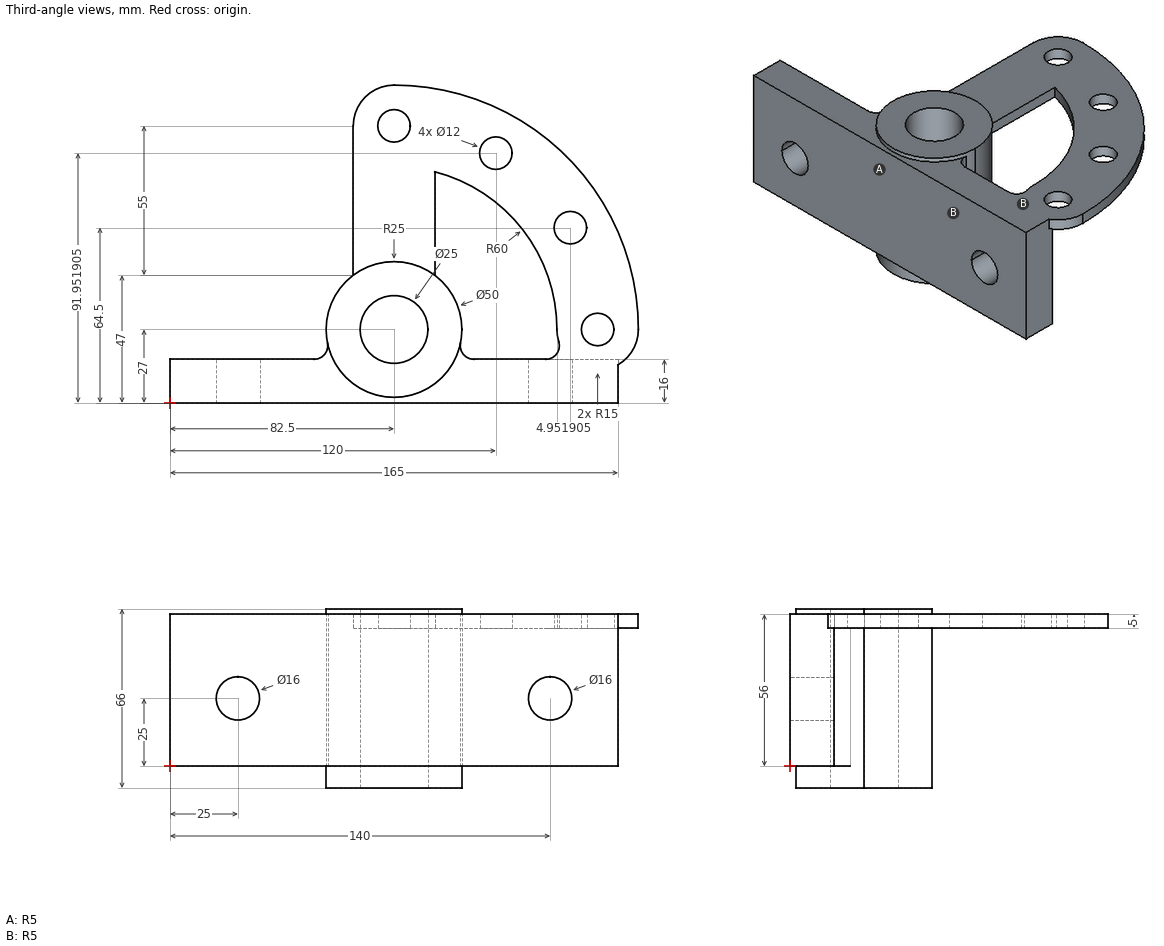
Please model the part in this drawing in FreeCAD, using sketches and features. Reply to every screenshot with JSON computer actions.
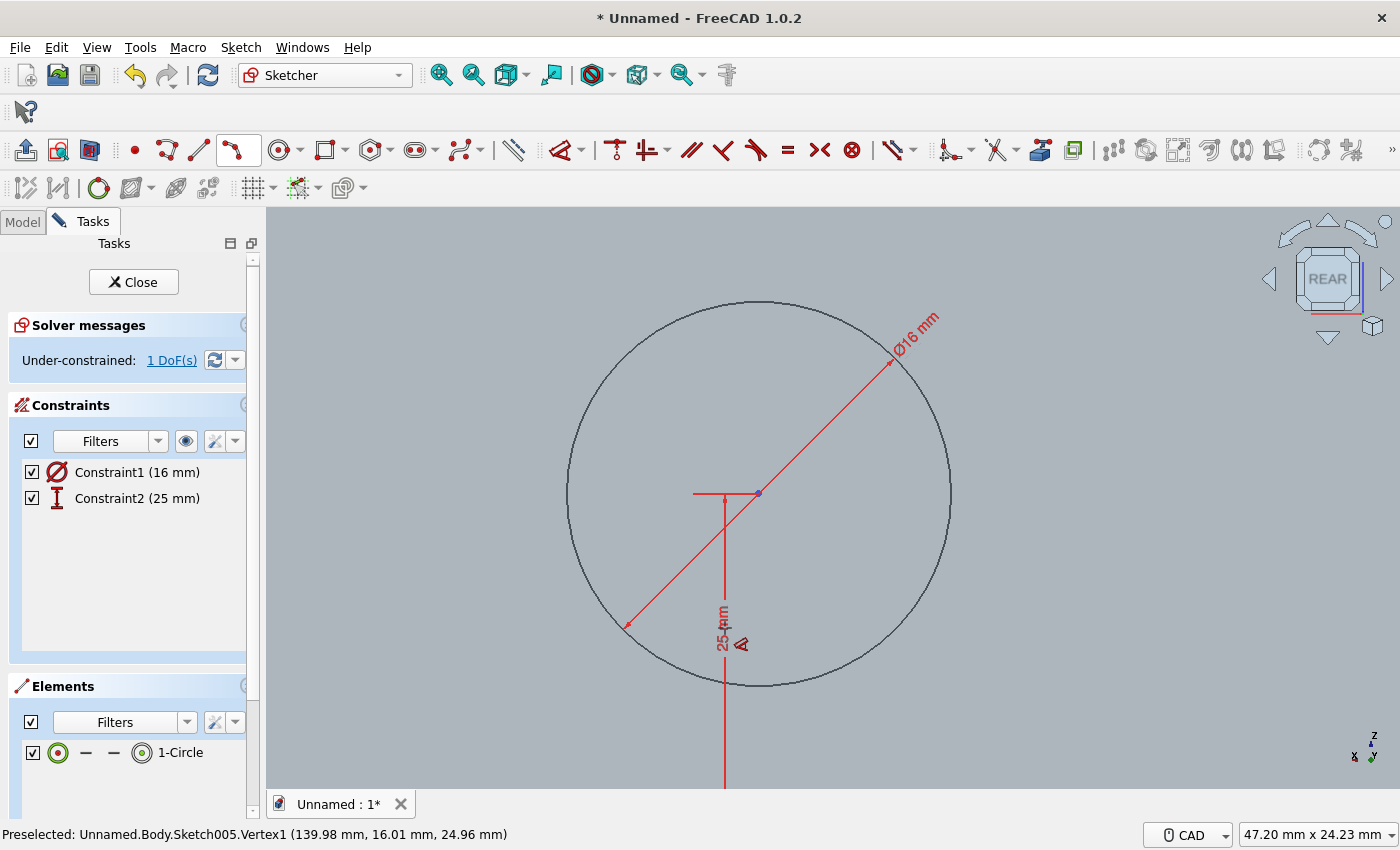
{"action": "left_click", "coordinate": [759, 494]}
{"action": "left_click", "coordinate": [997, 460]}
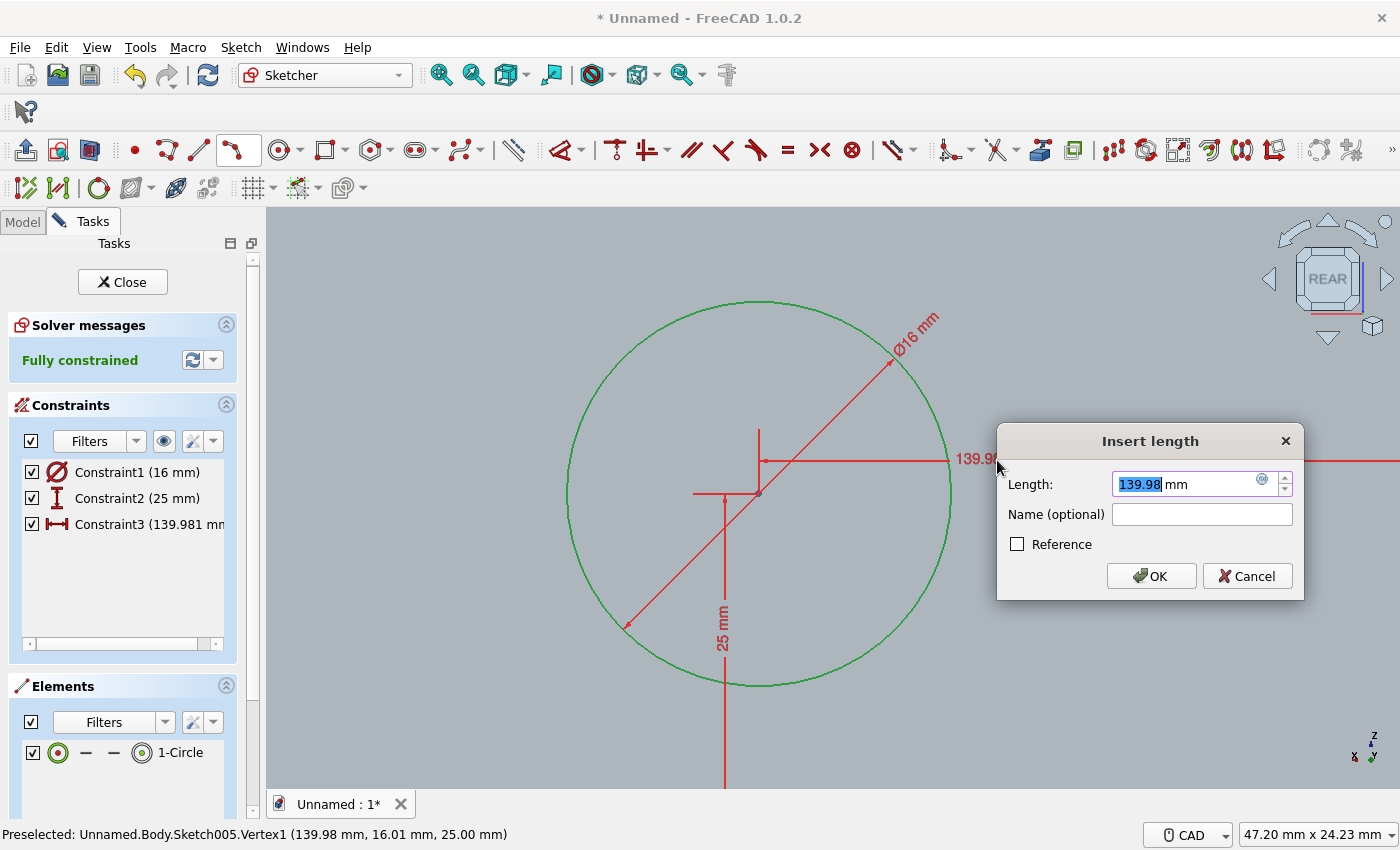
{"action": "type", "text": "140"}
{"action": "key", "text": "Return"}
{"action": "key", "text": "Escape"}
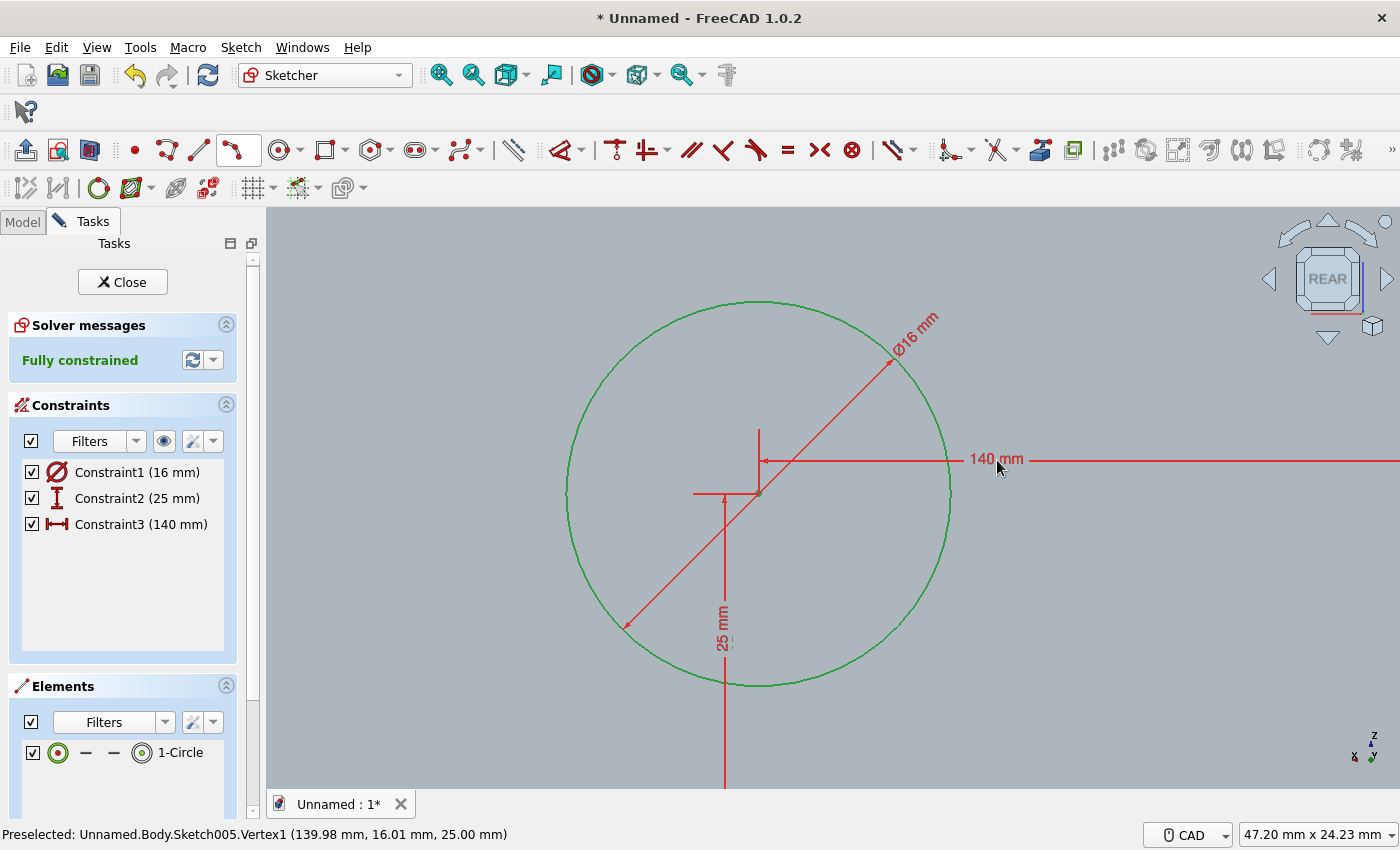
{"action": "left_click", "coordinate": [123, 282]}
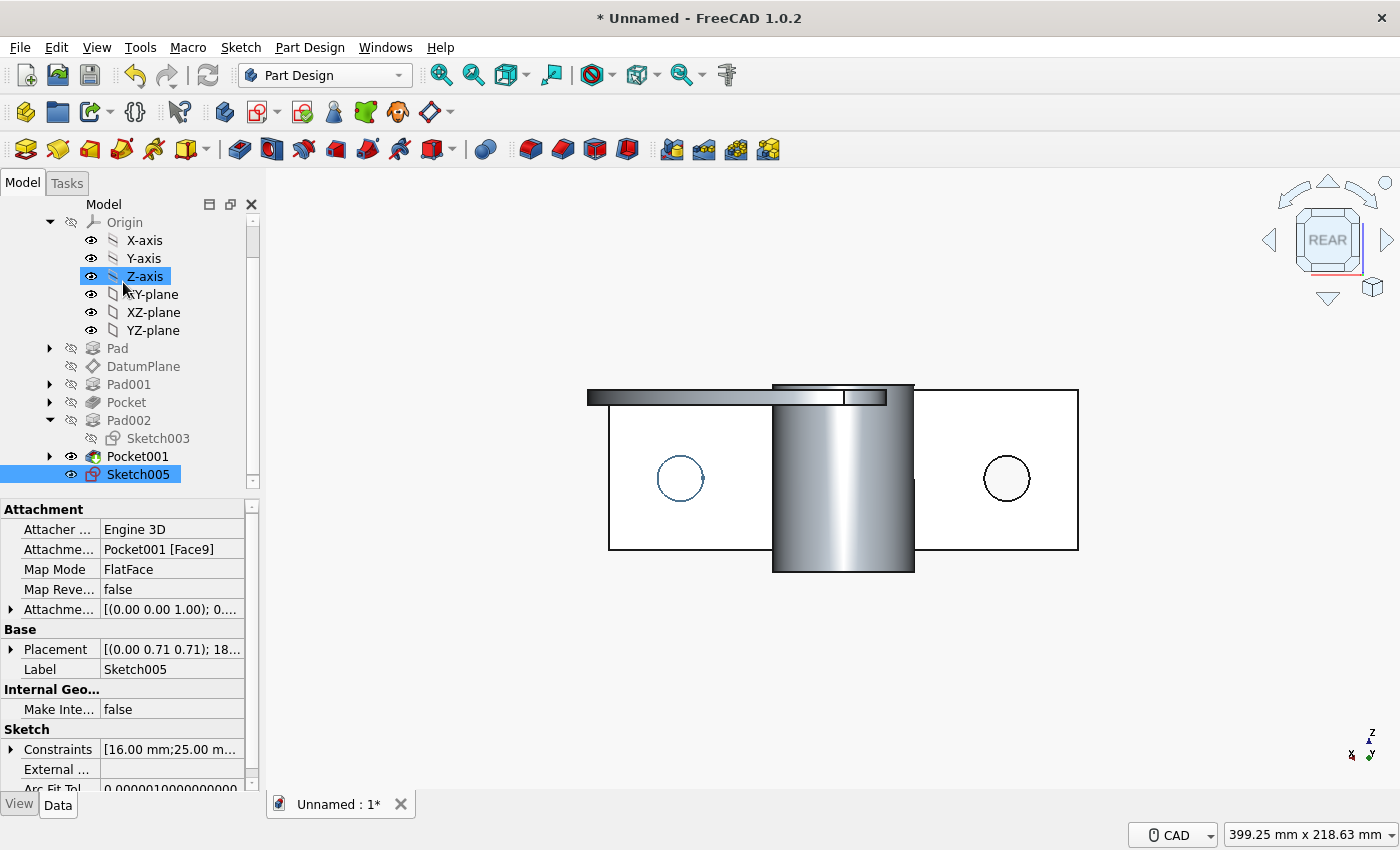
{"action": "left_click", "coordinate": [240, 150]}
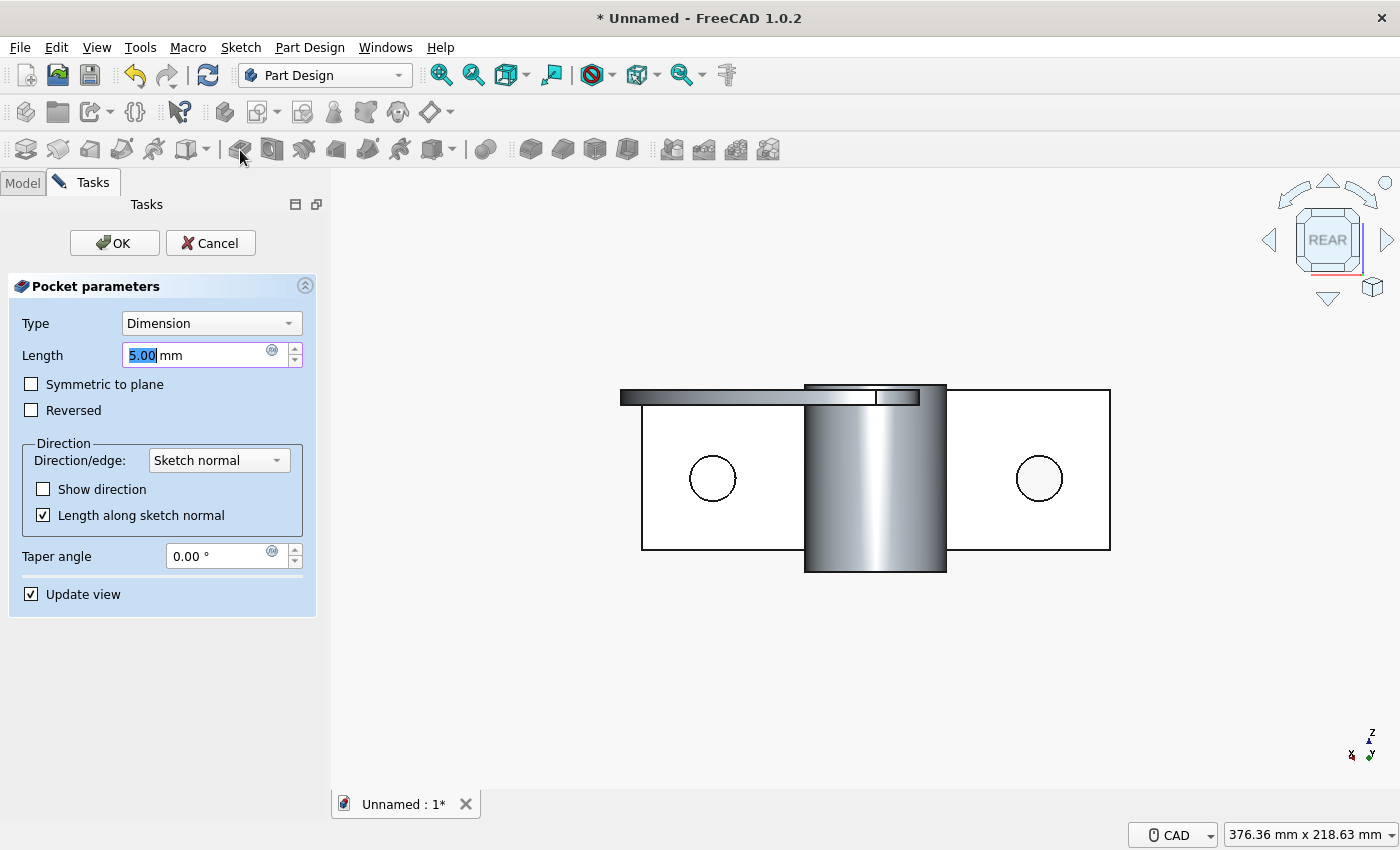
{"action": "left_click", "coordinate": [212, 324]}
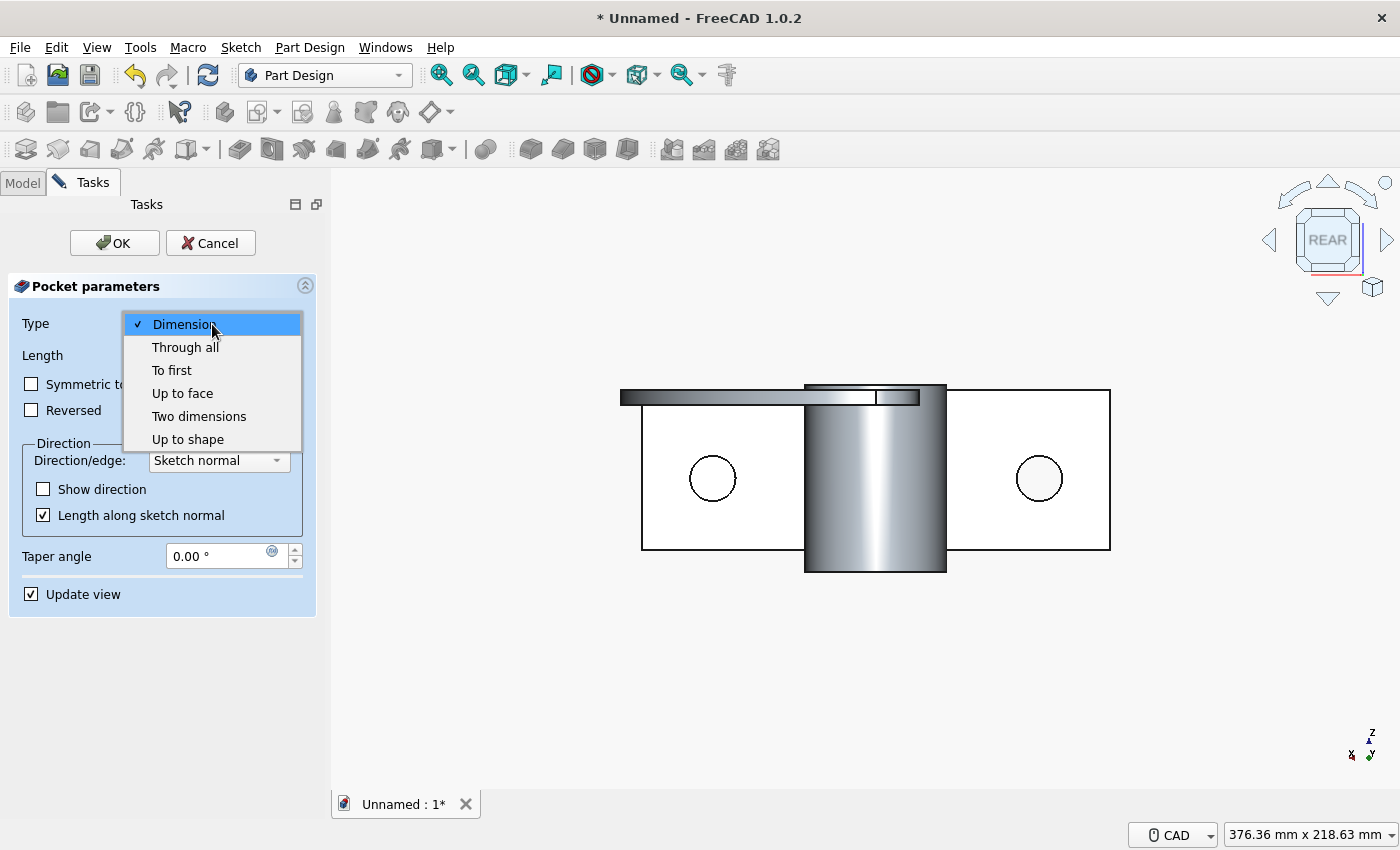
{"action": "left_click", "coordinate": [212, 348]}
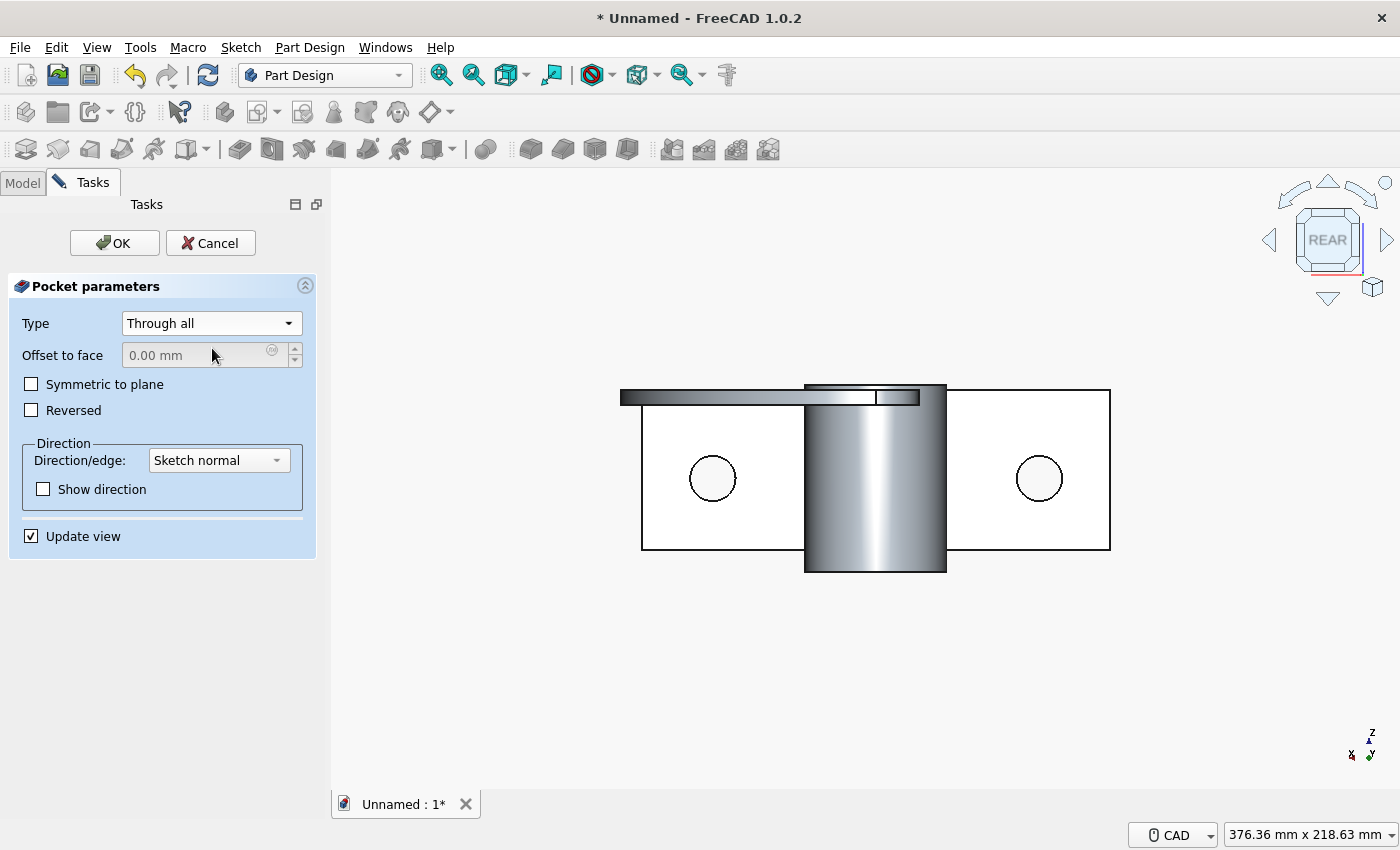
{"action": "left_click", "coordinate": [115, 243]}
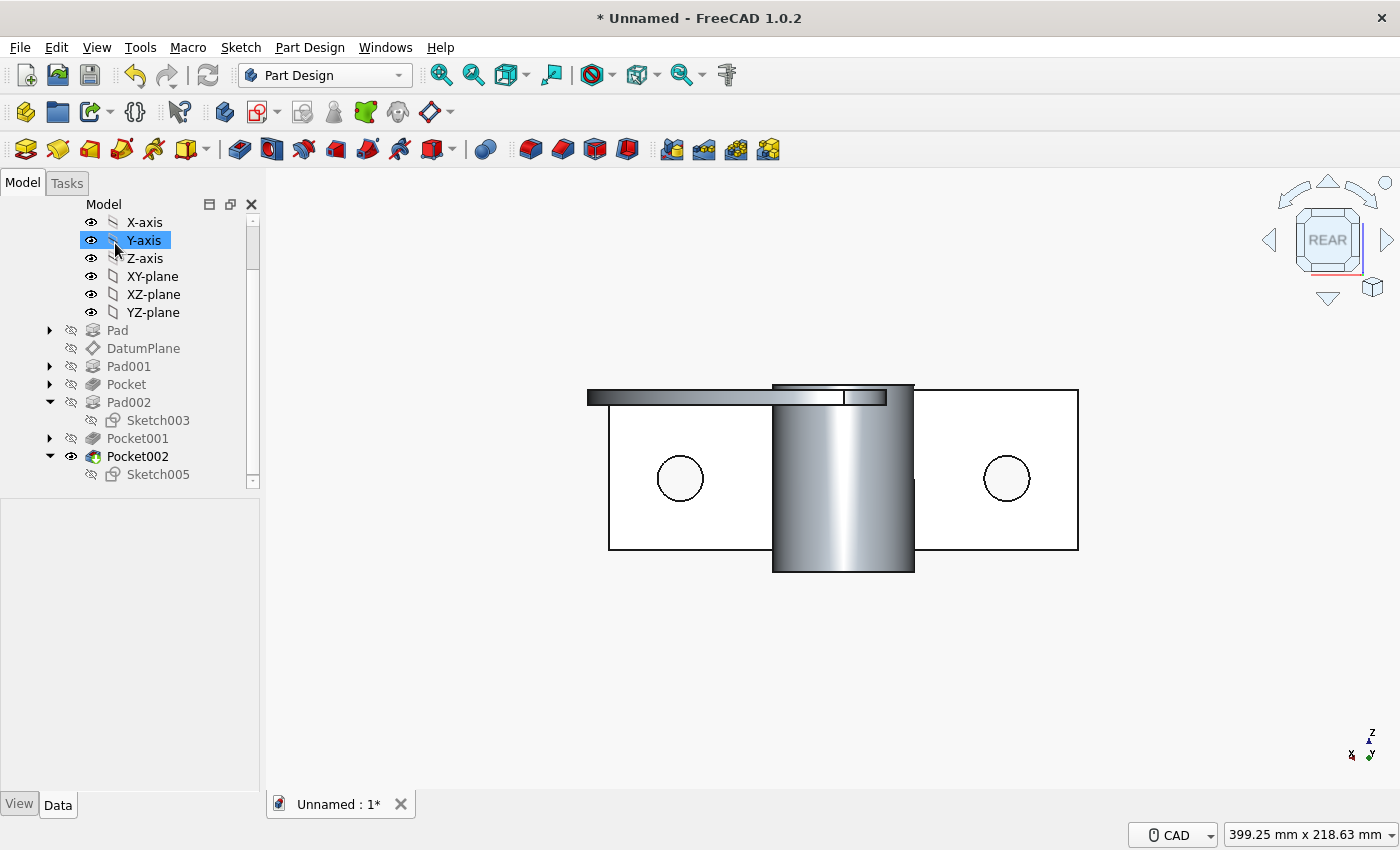
{"action": "left_click", "coordinate": [442, 76]}